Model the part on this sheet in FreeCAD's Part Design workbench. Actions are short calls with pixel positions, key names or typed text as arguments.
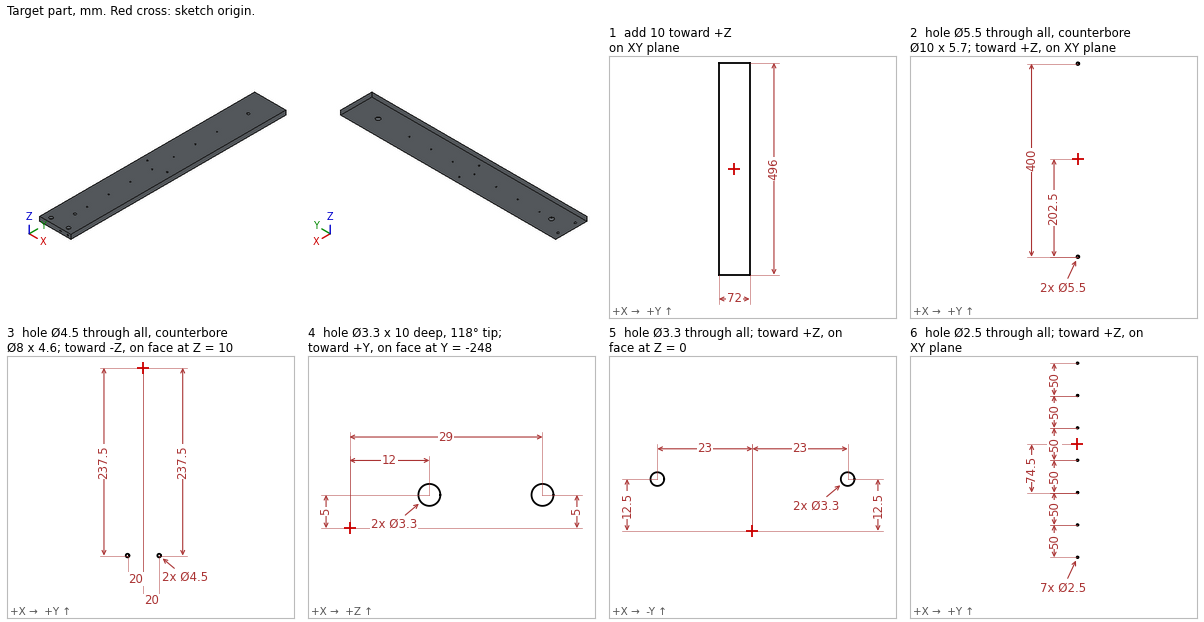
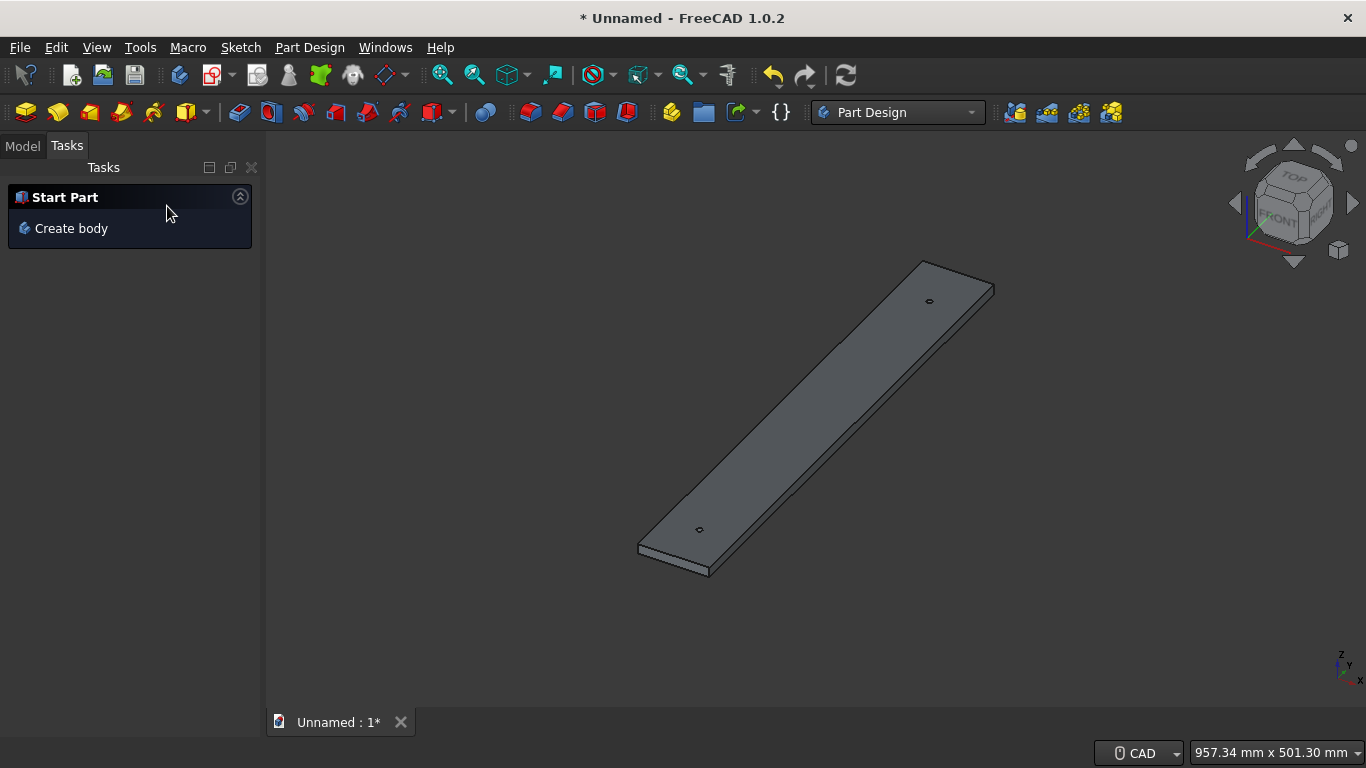
click(897, 332)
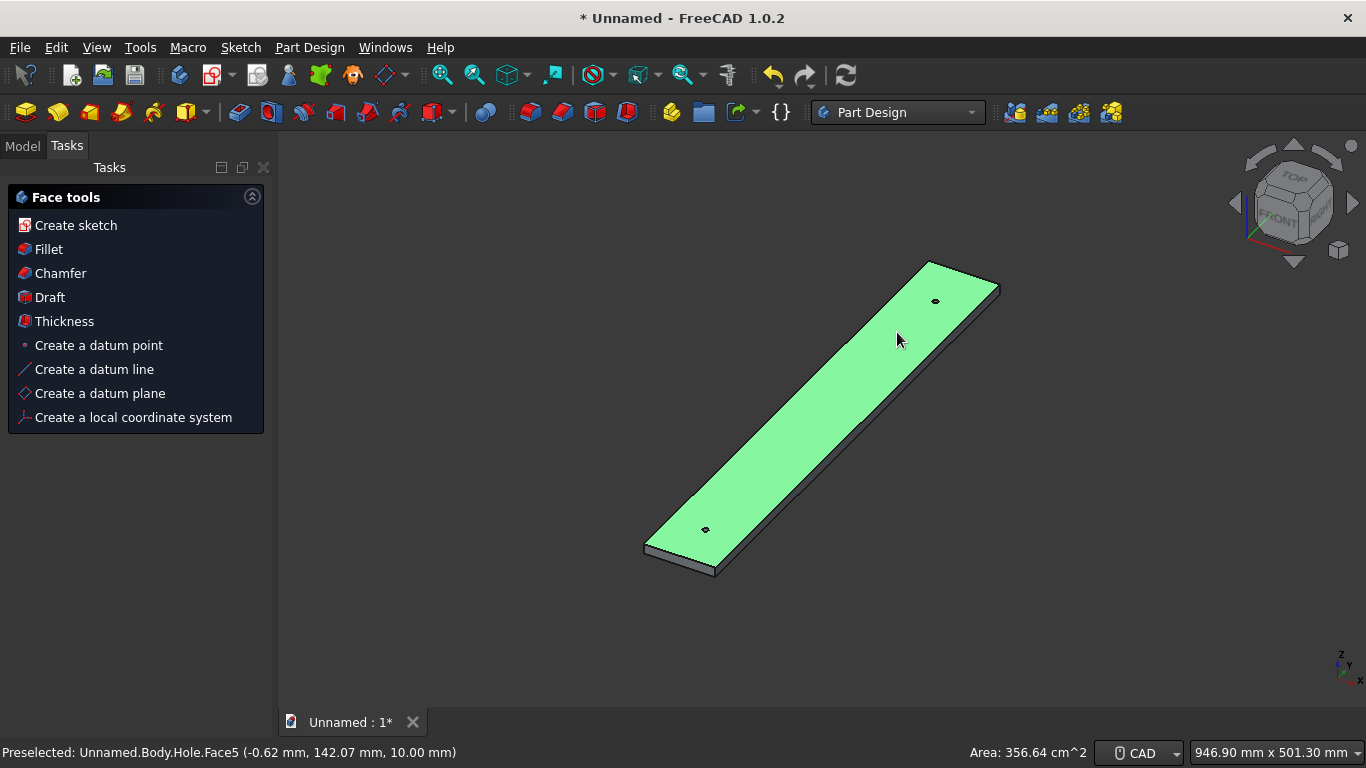
click(212, 76)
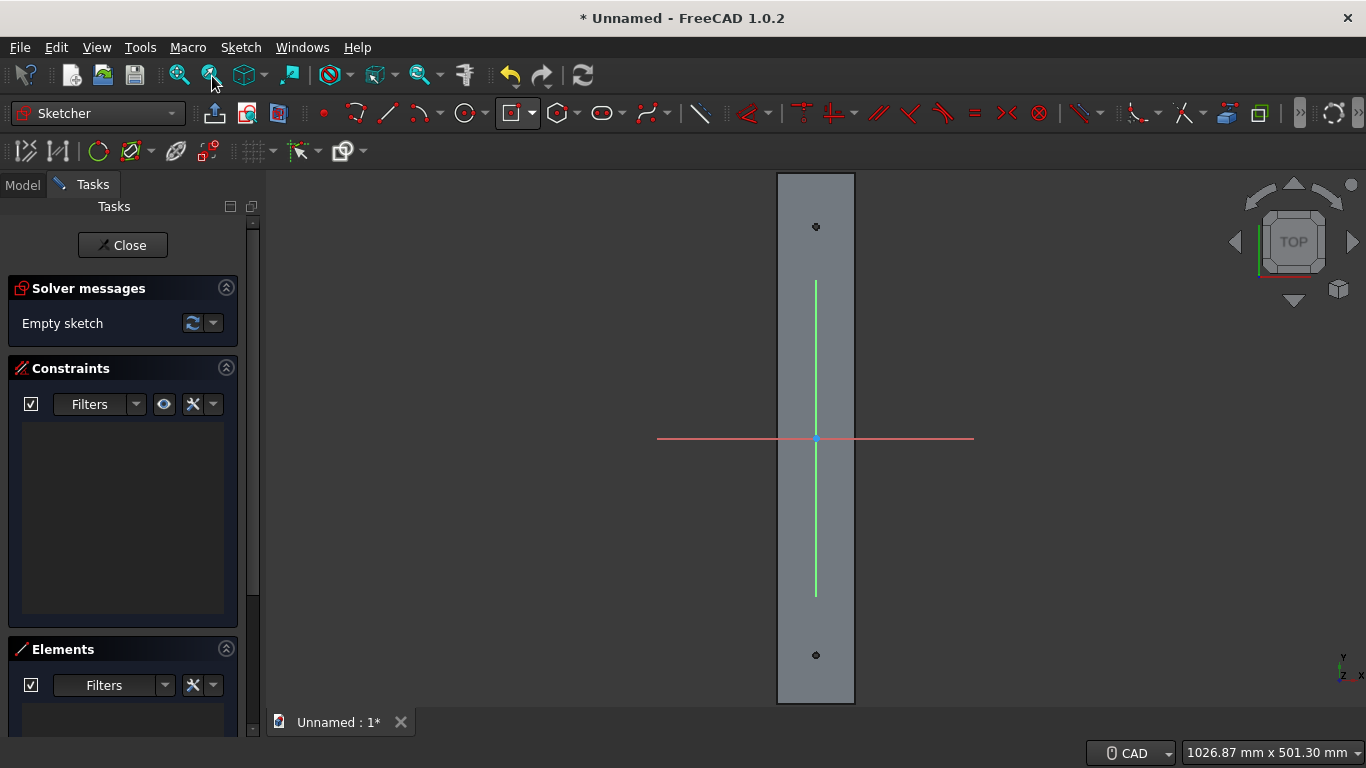
scroll(748, 438, down, 5)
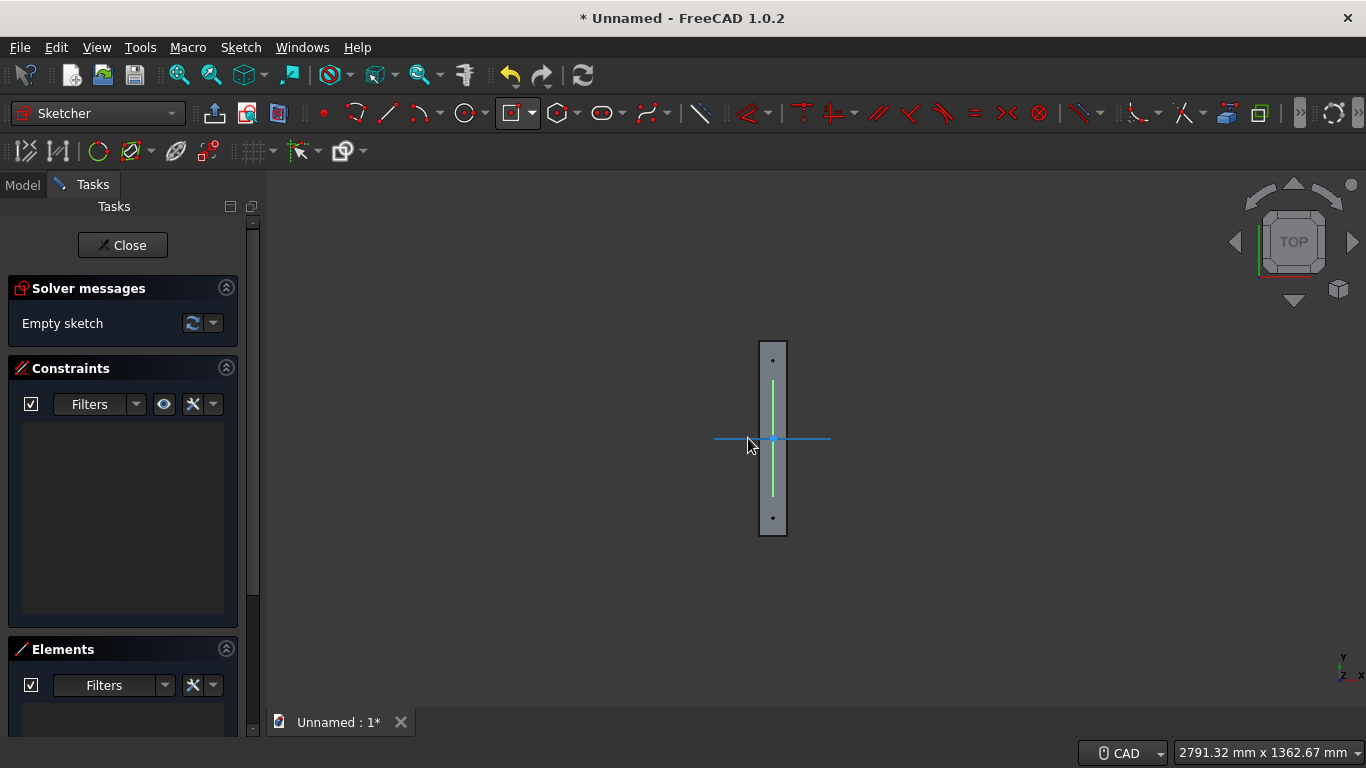
scroll(775, 537, up, 15)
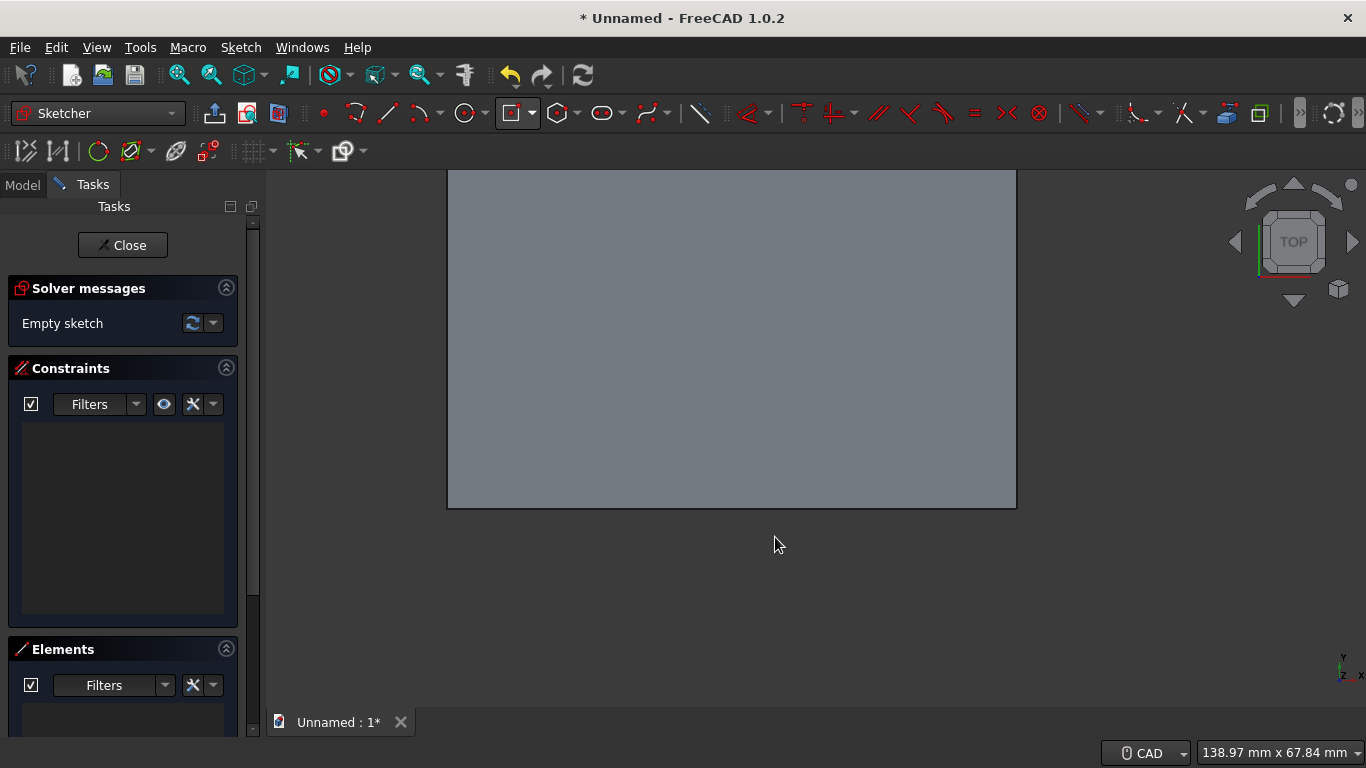
scroll(713, 409, up, 3)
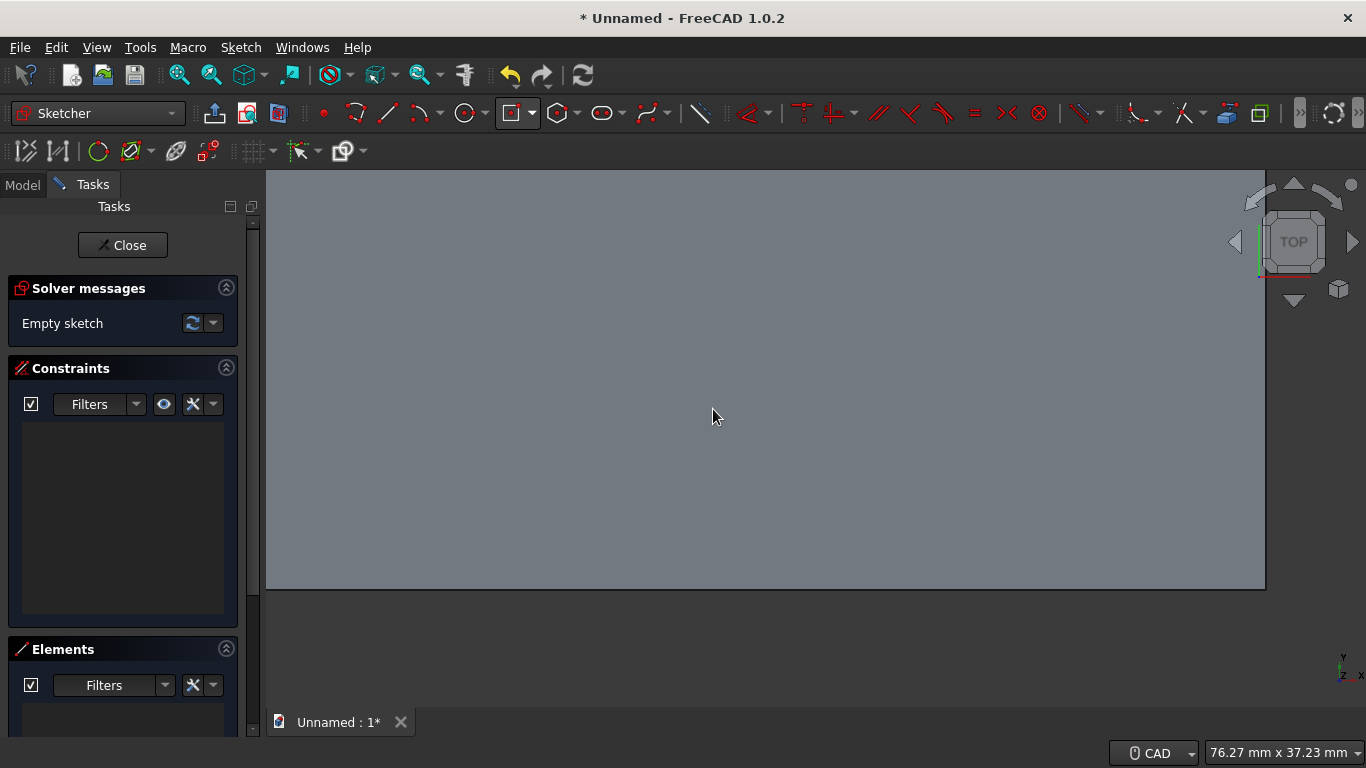
click(466, 114)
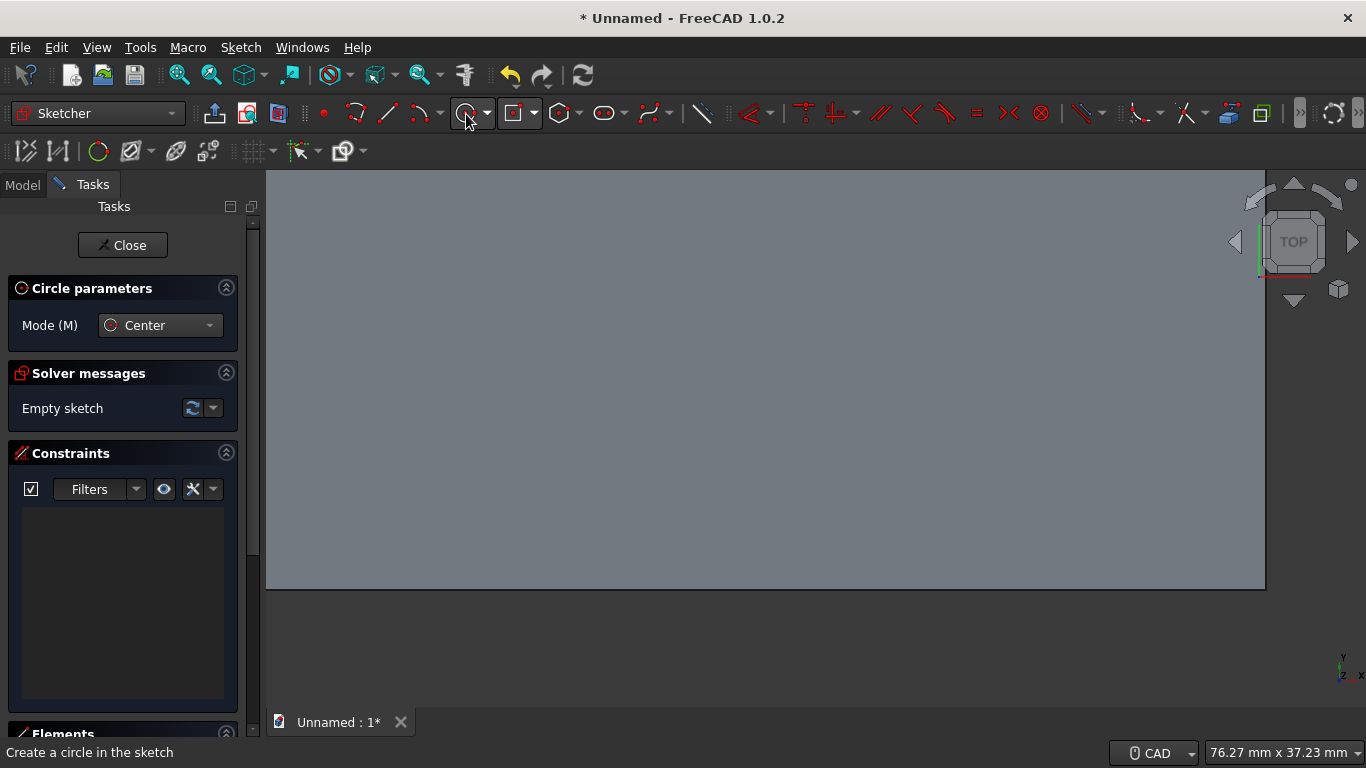
click(459, 438)
click(482, 416)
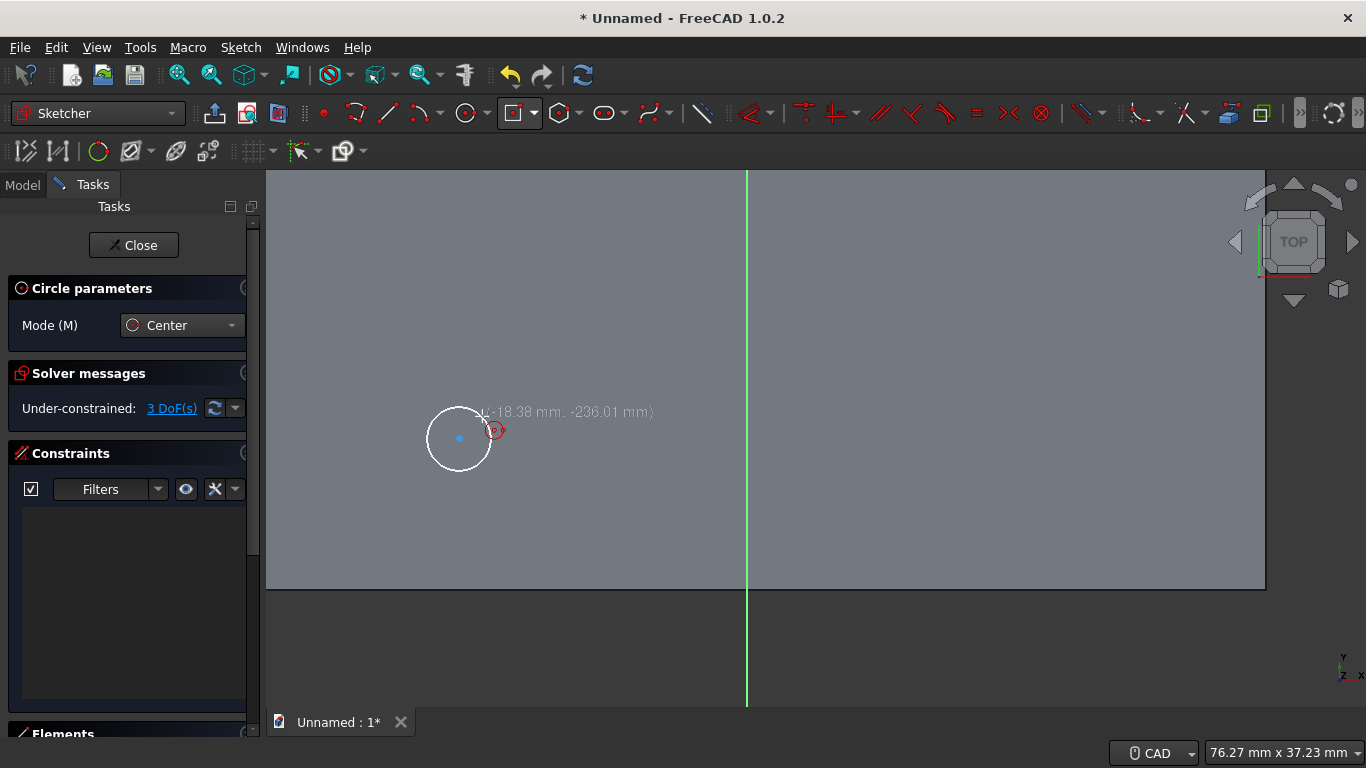
click(1036, 438)
click(1058, 416)
key(Escape)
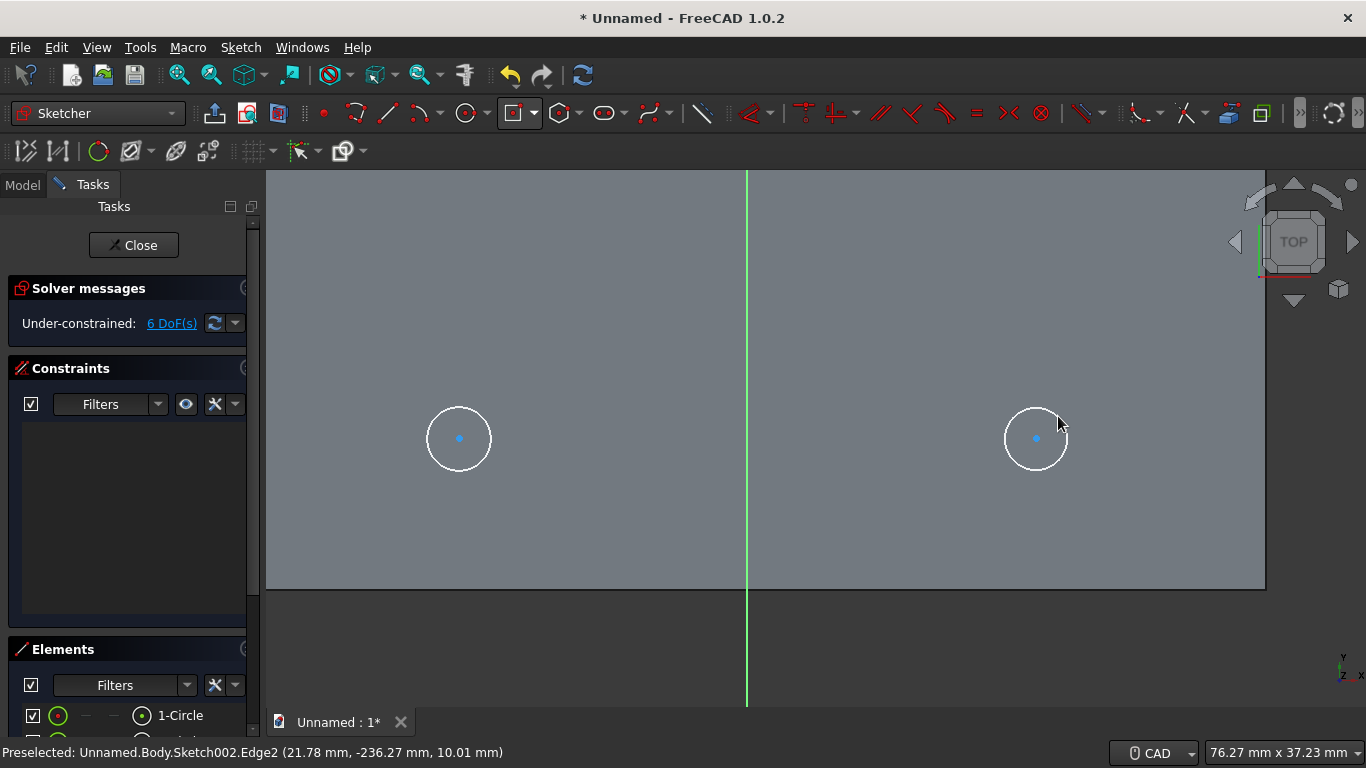
click(481, 416)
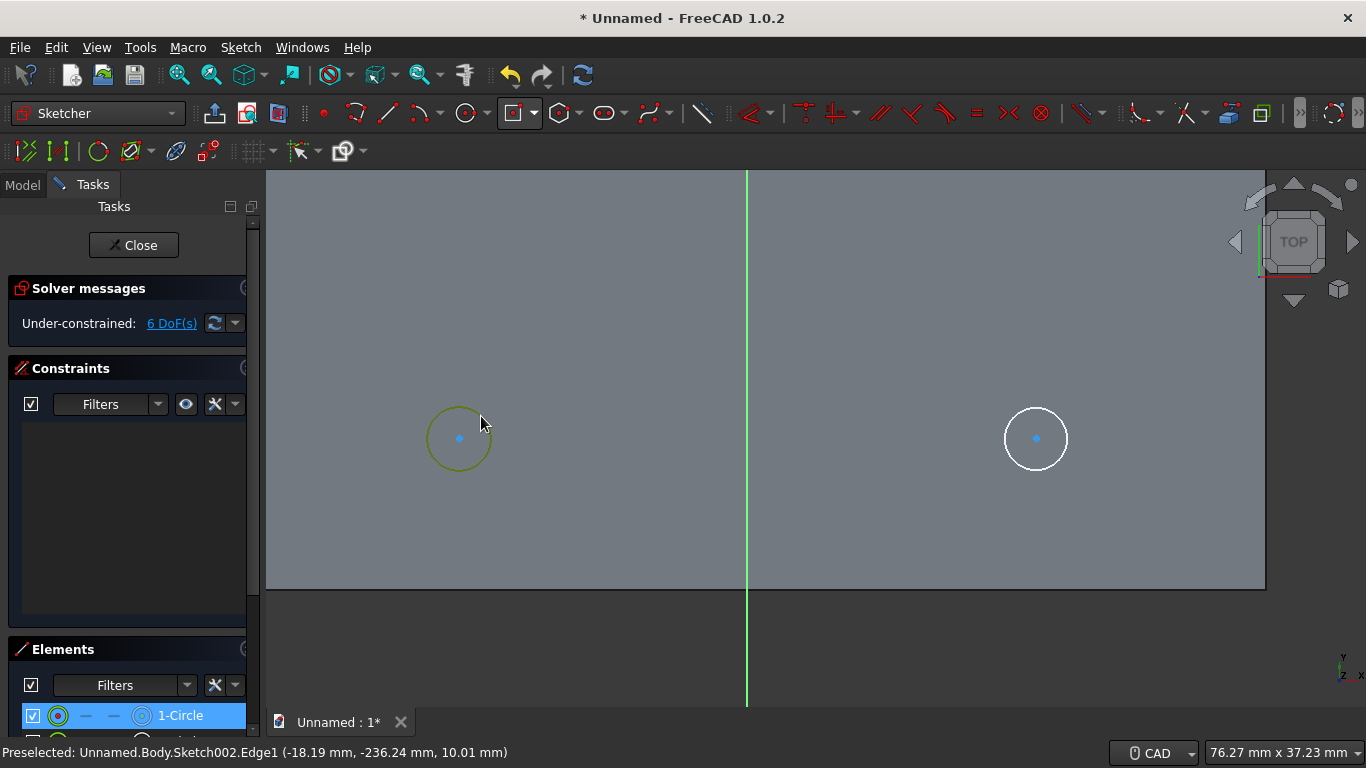
click(1058, 417)